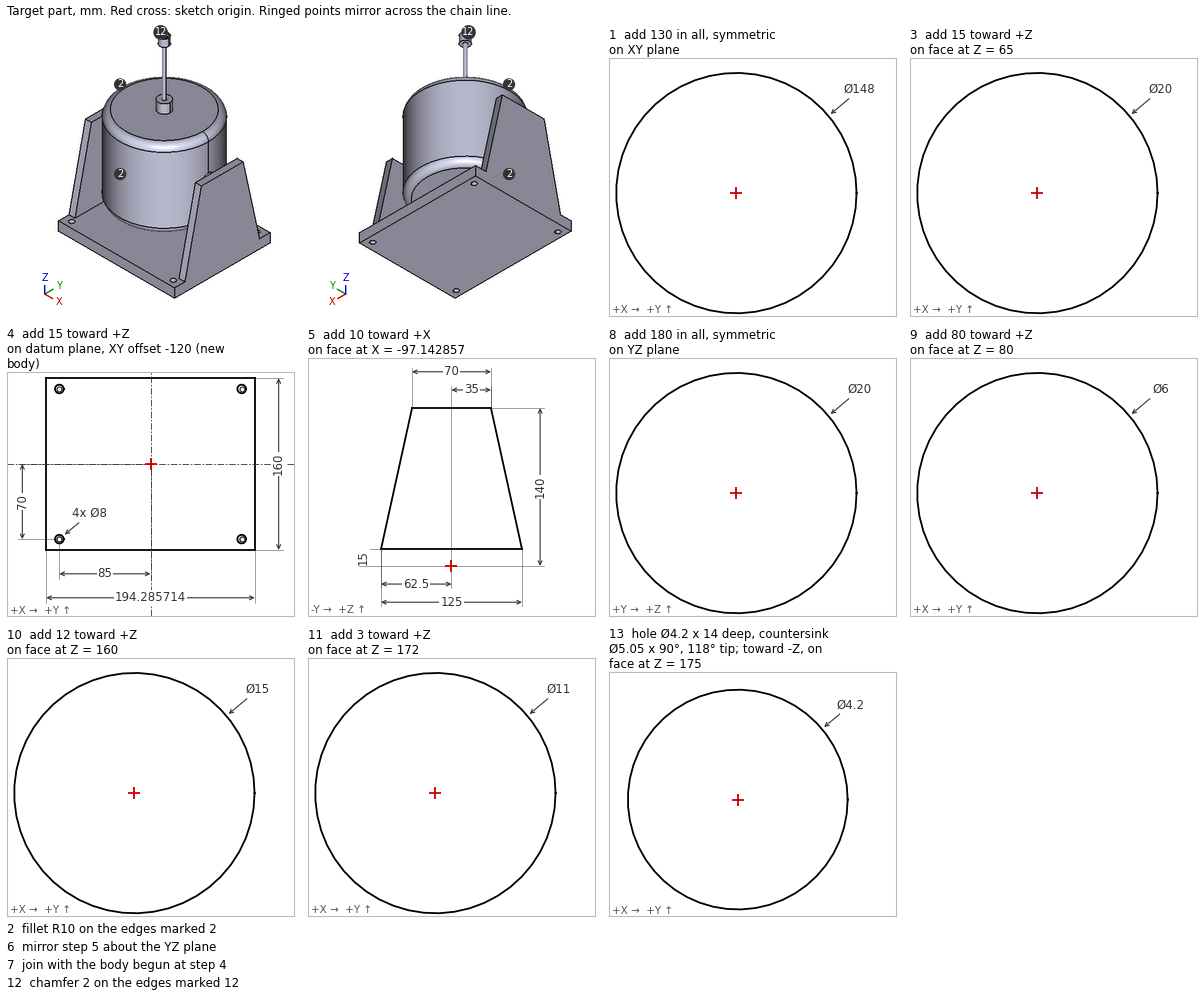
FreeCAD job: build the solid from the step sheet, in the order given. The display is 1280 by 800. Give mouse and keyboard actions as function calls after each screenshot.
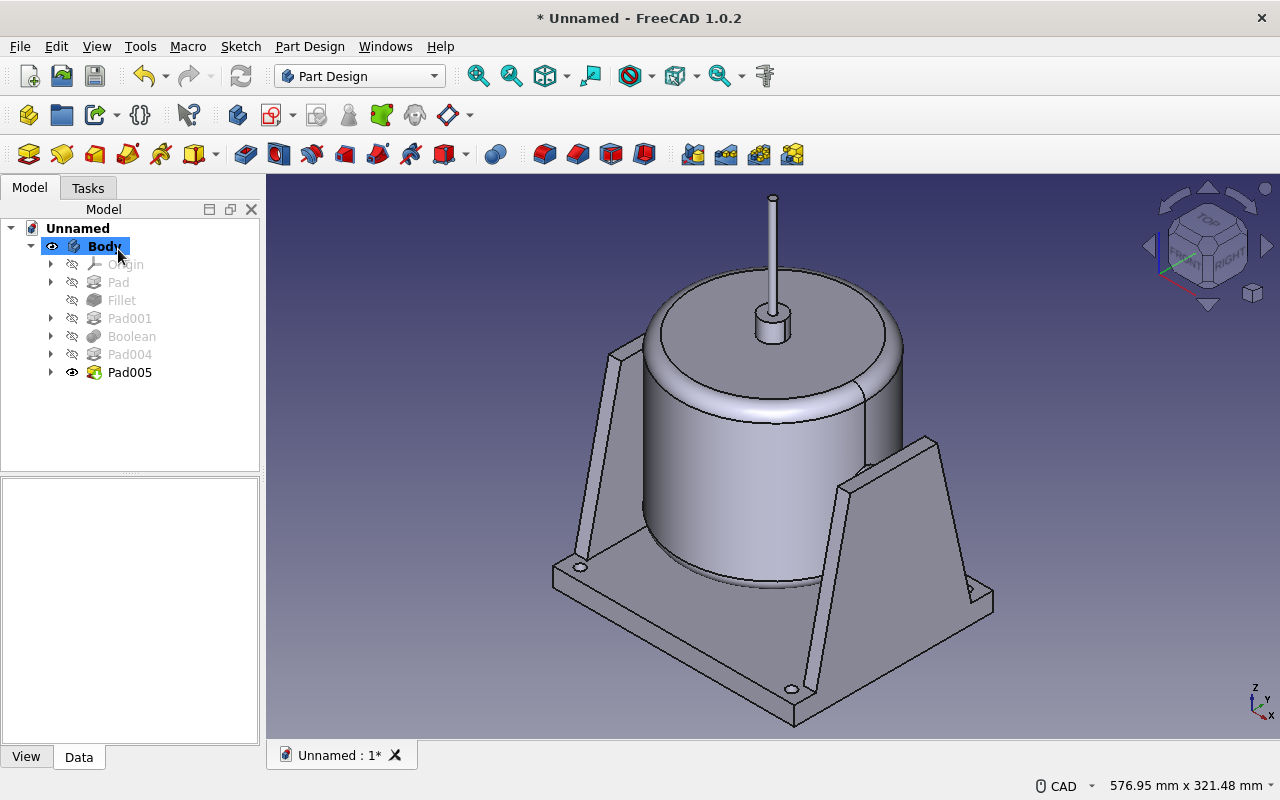
click(479, 76)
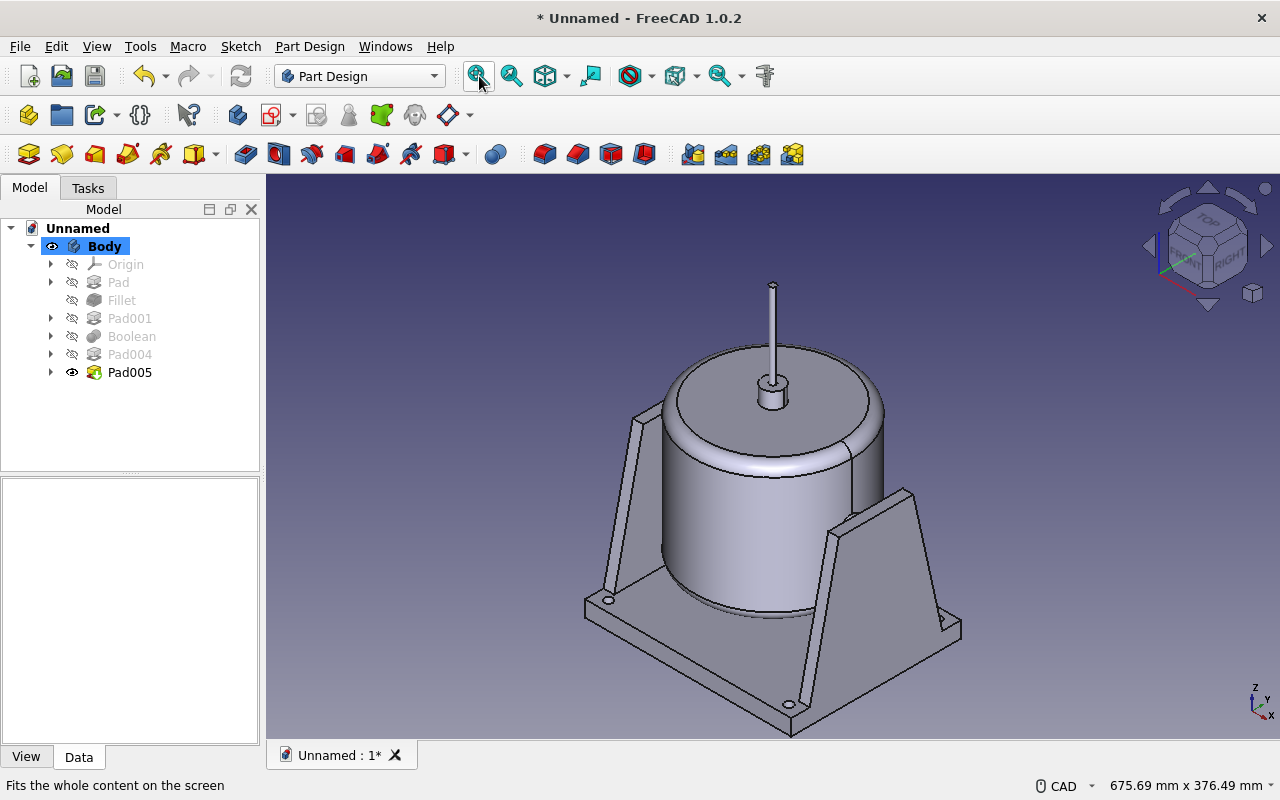
scroll(773, 284, up, 5)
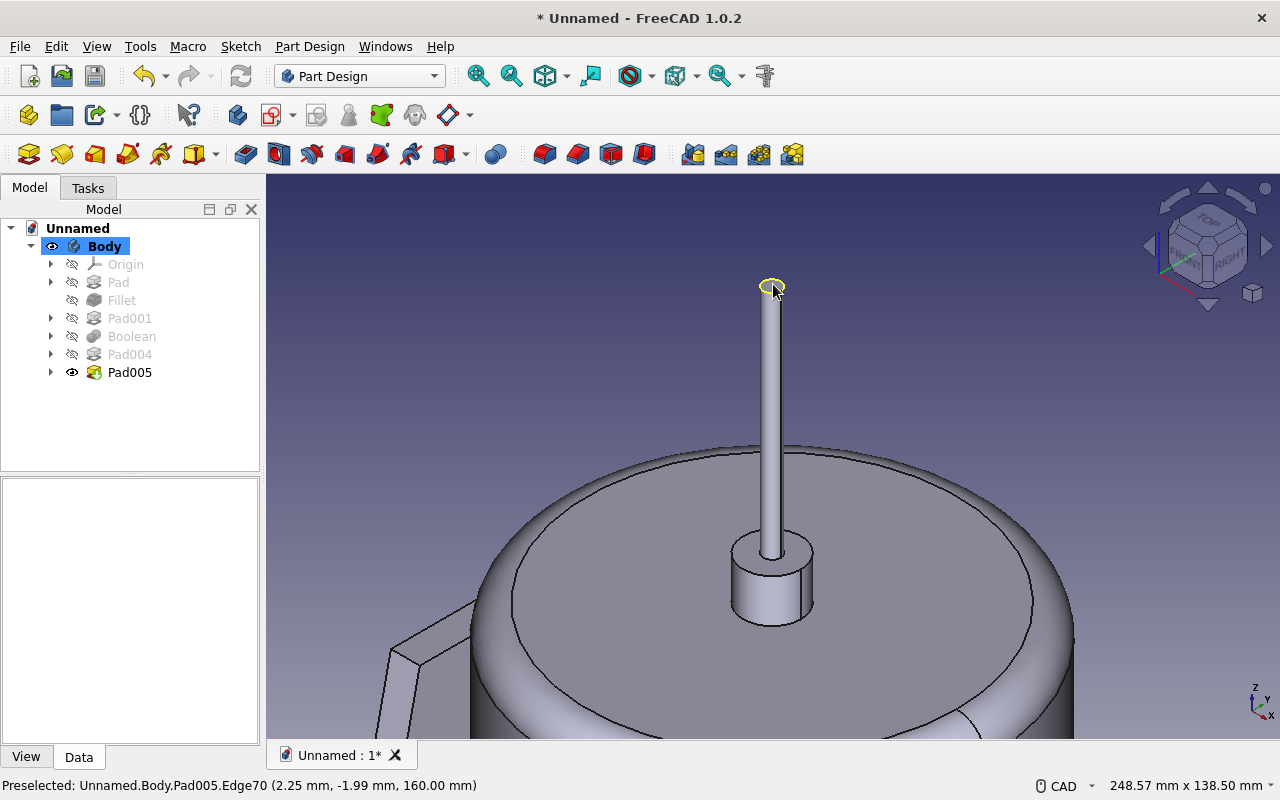
key(v)
key(f)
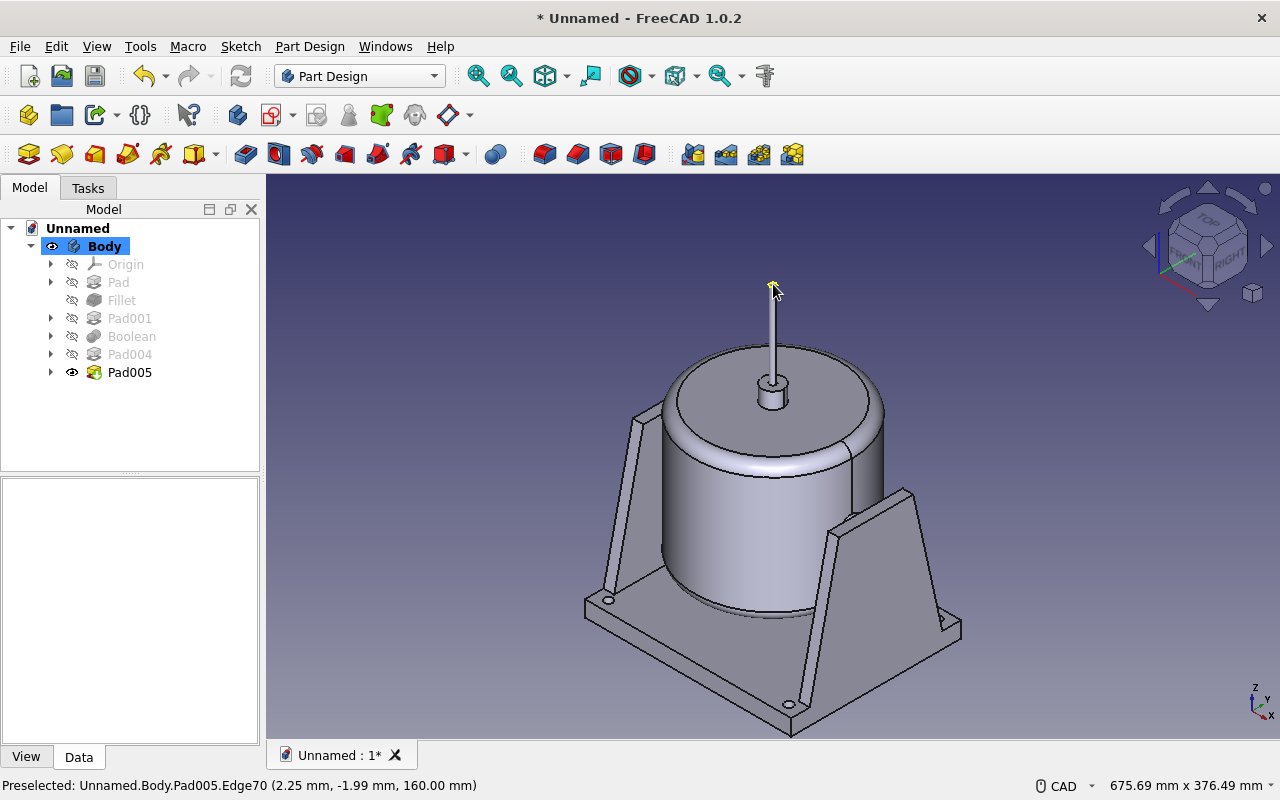
key(2)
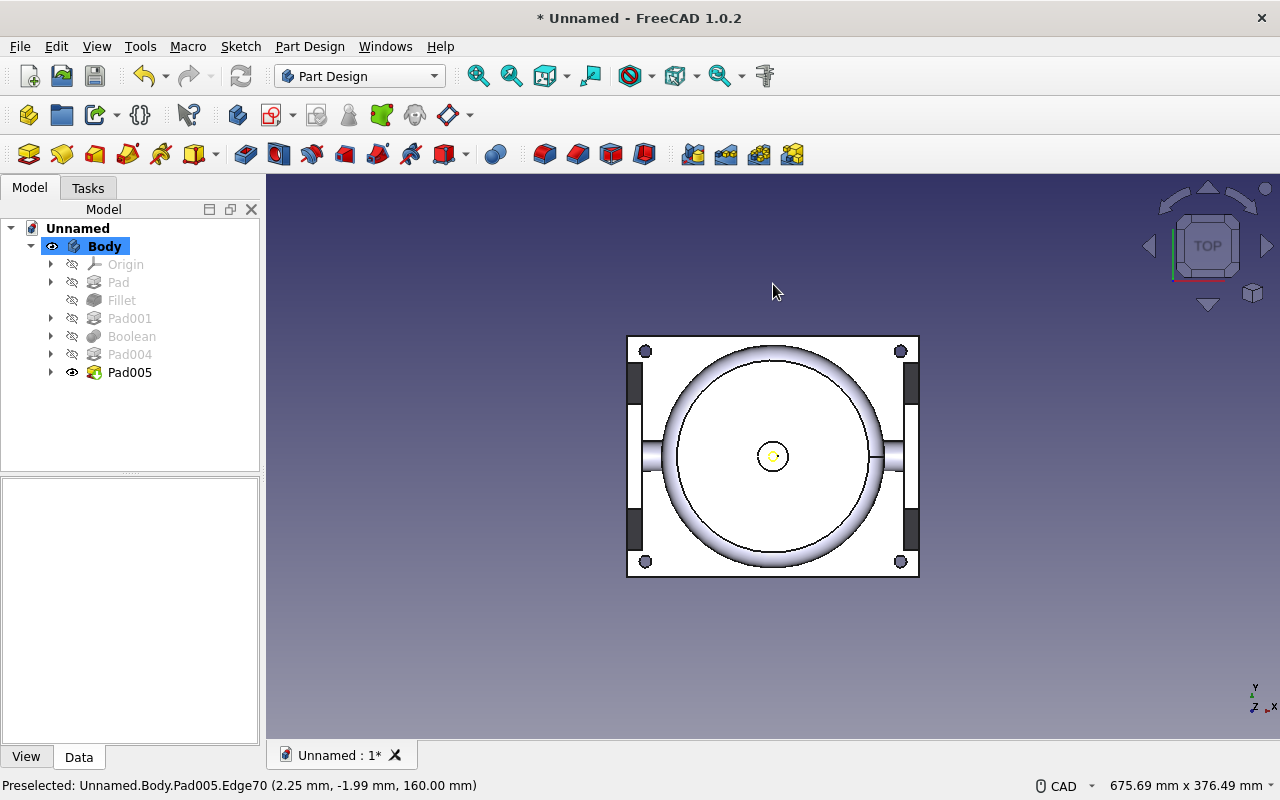
key(v)
key(f)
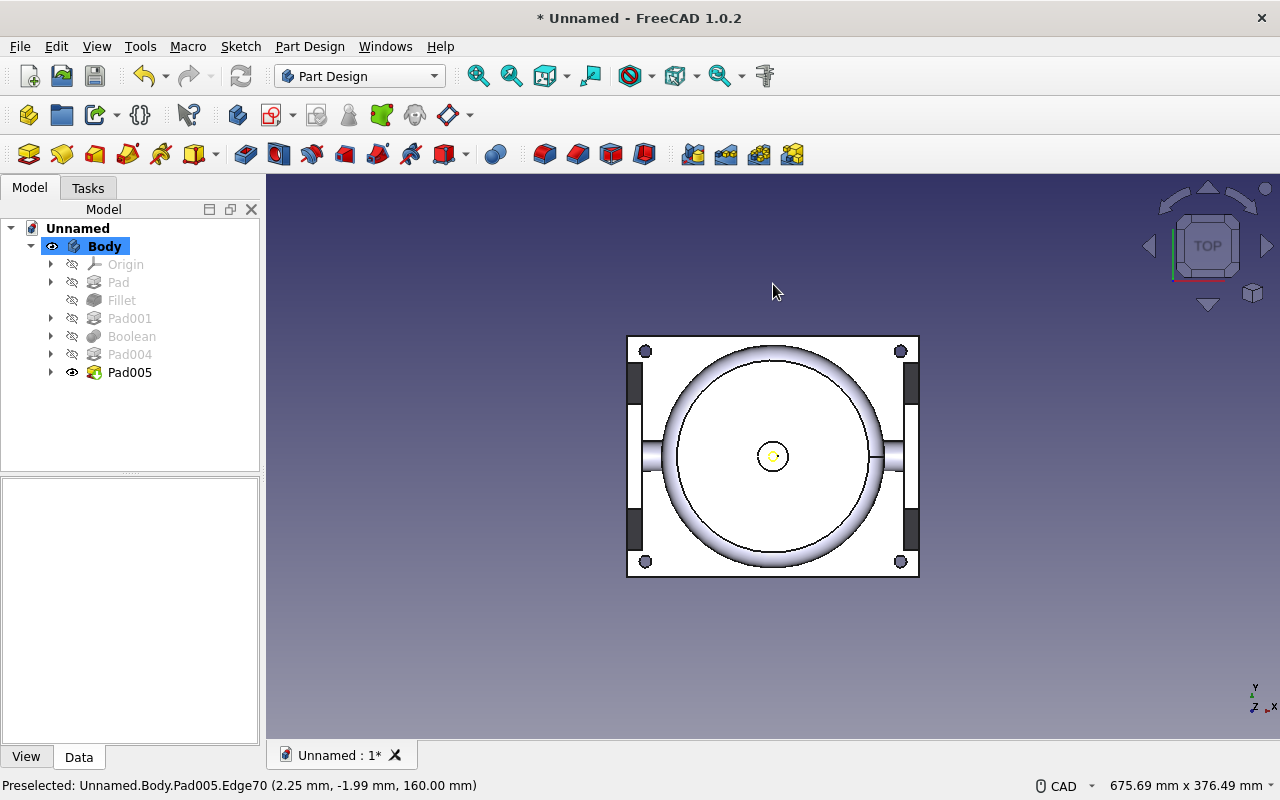
scroll(773, 455, up, 5)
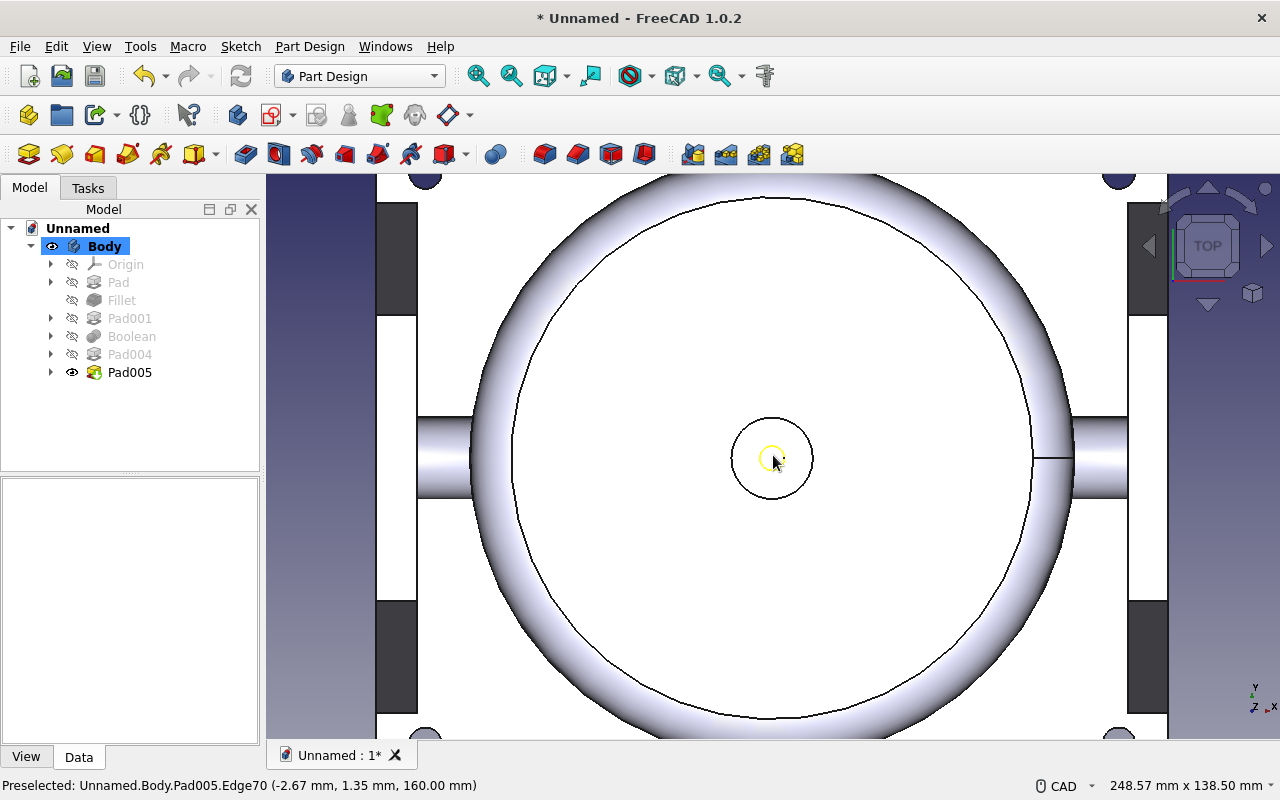
click(772, 457)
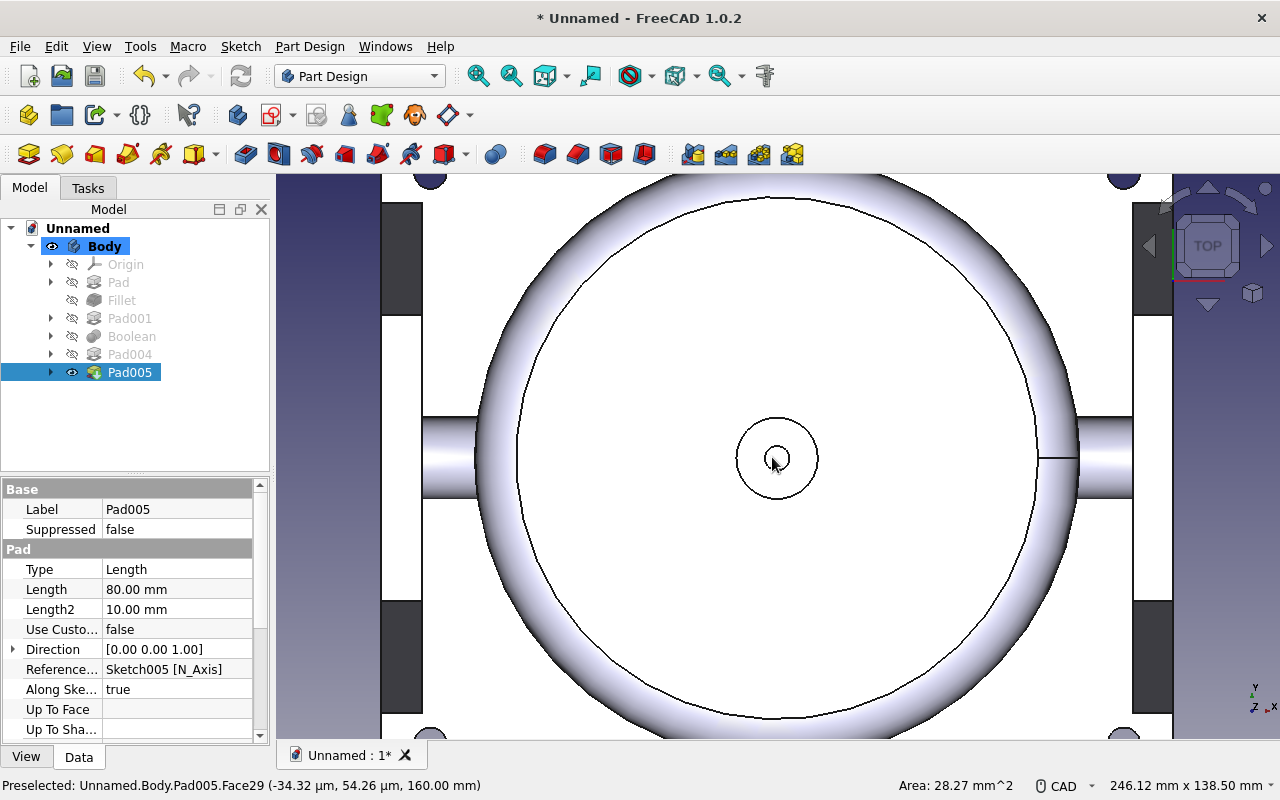
click(270, 116)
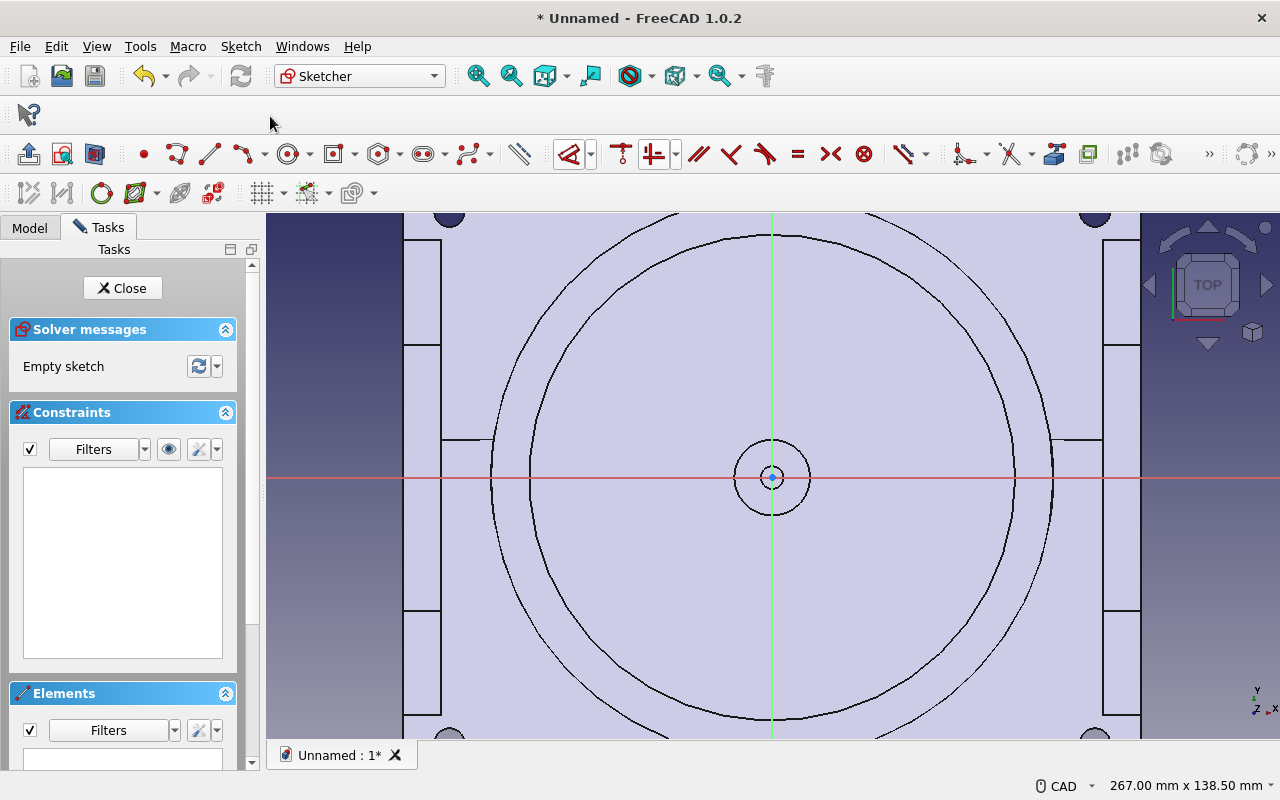
scroll(786, 478, up, 9)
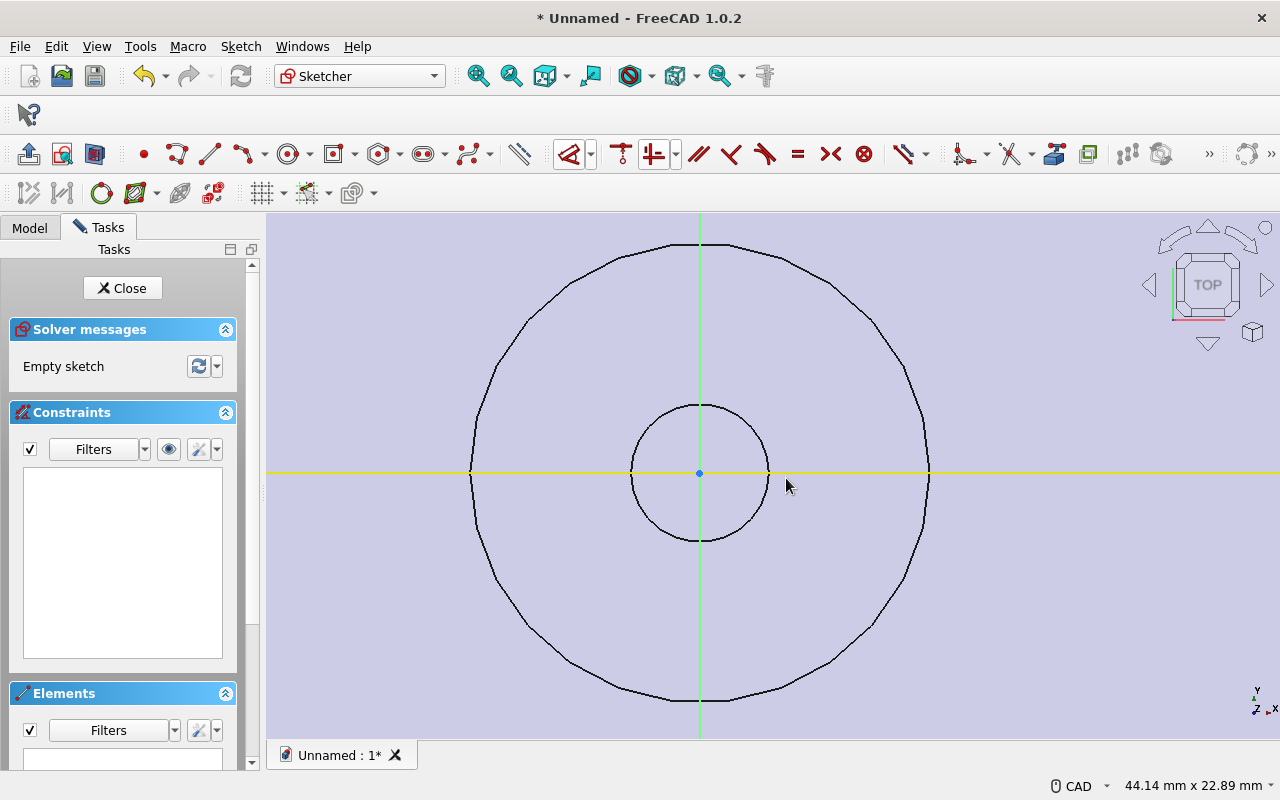
key(g)
key(c)